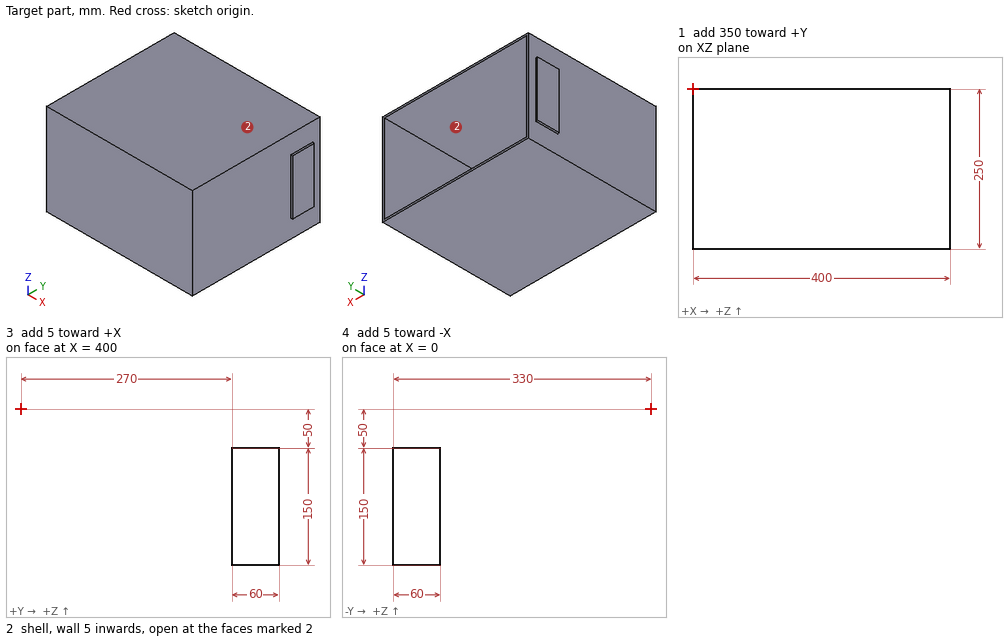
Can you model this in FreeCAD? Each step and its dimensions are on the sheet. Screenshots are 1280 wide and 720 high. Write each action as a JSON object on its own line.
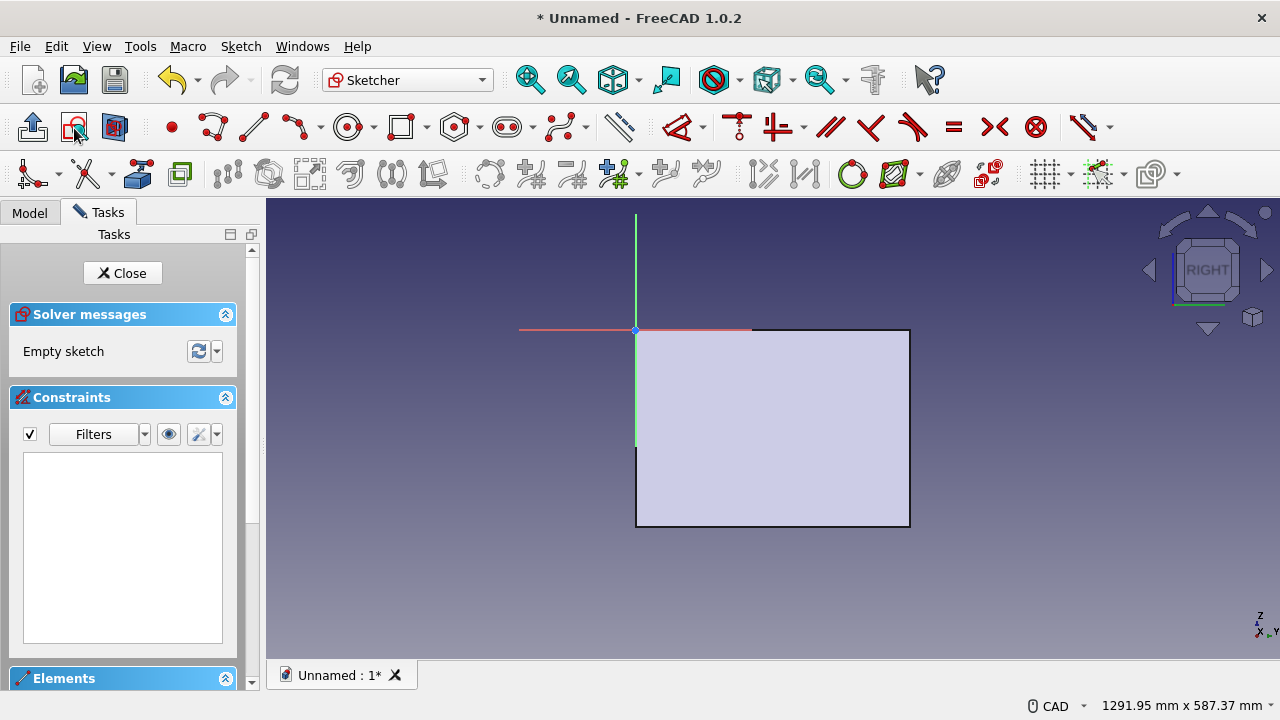
{"action": "scroll", "coordinate": [839, 385], "scroll_direction": "up", "scroll_amount": 3}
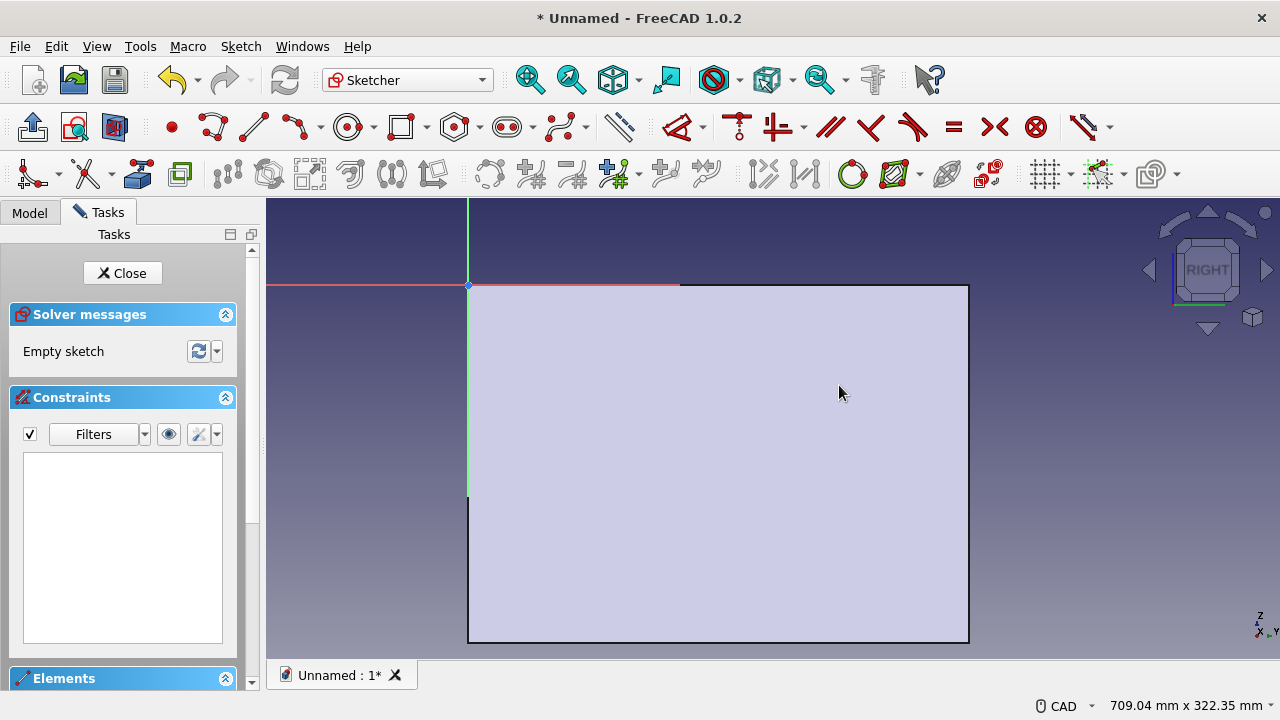
{"action": "left_click", "coordinate": [400, 128]}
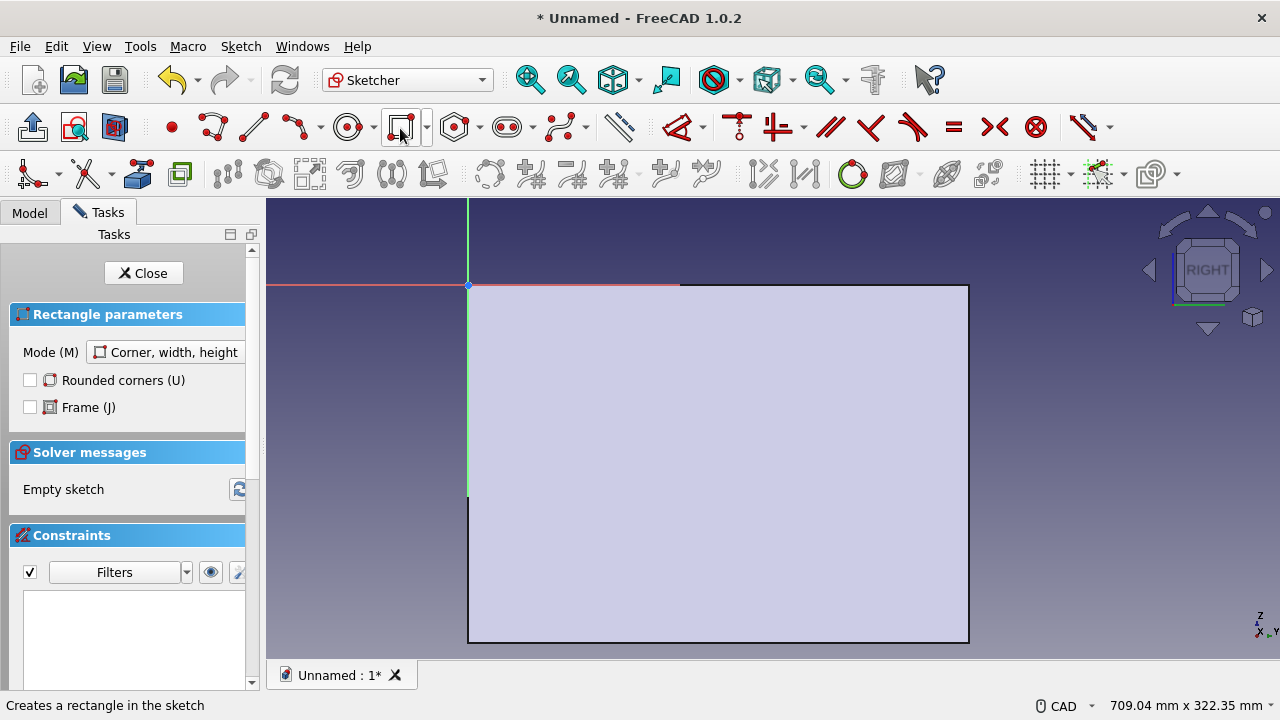
{"action": "left_click", "coordinate": [854, 357]}
{"action": "mouse_move", "coordinate": [940, 571]}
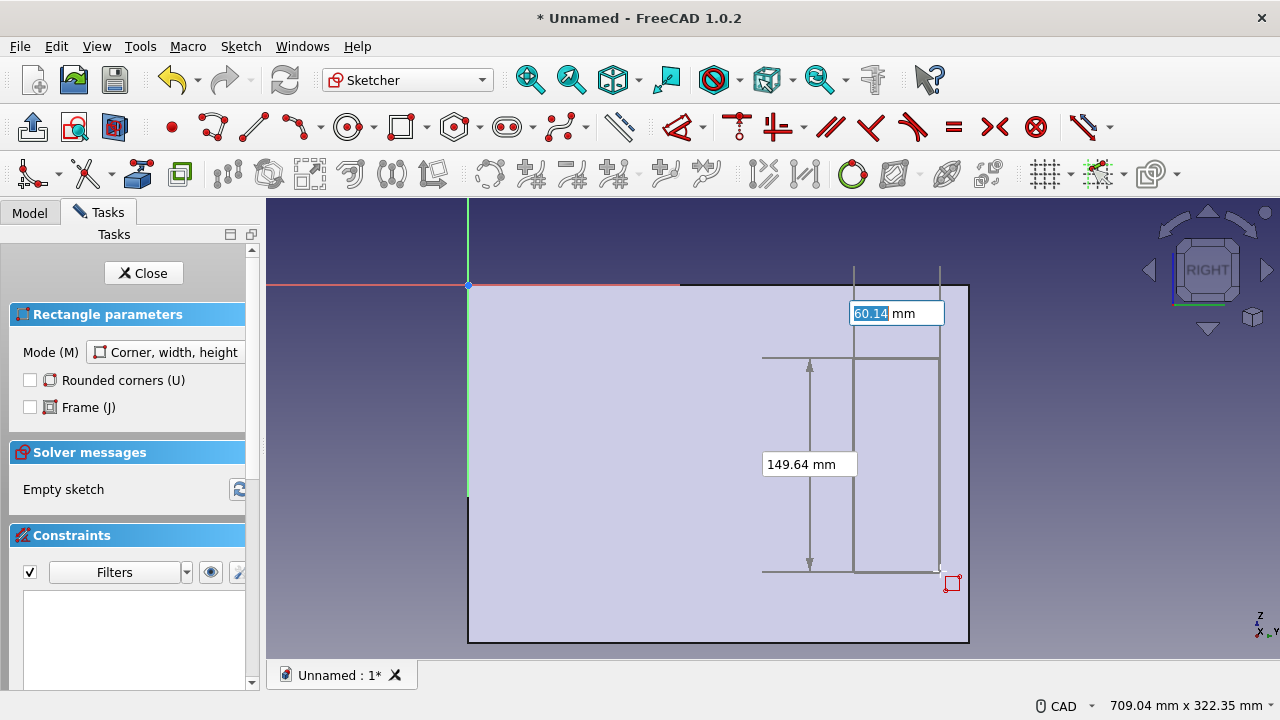
{"action": "type", "text": "60"}
{"action": "key", "text": "Tab"}
{"action": "type", "text": "150"}
{"action": "key", "text": "Return"}
{"action": "key", "text": "Escape"}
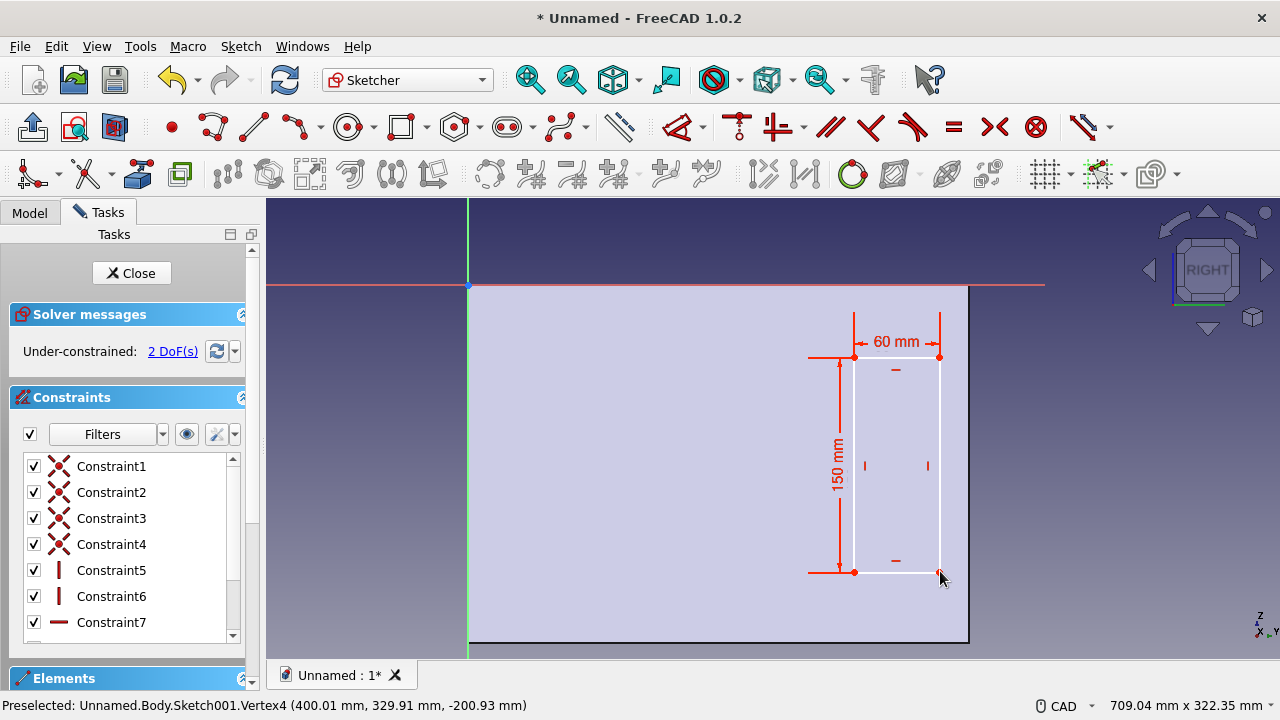
{"action": "key", "text": "d"}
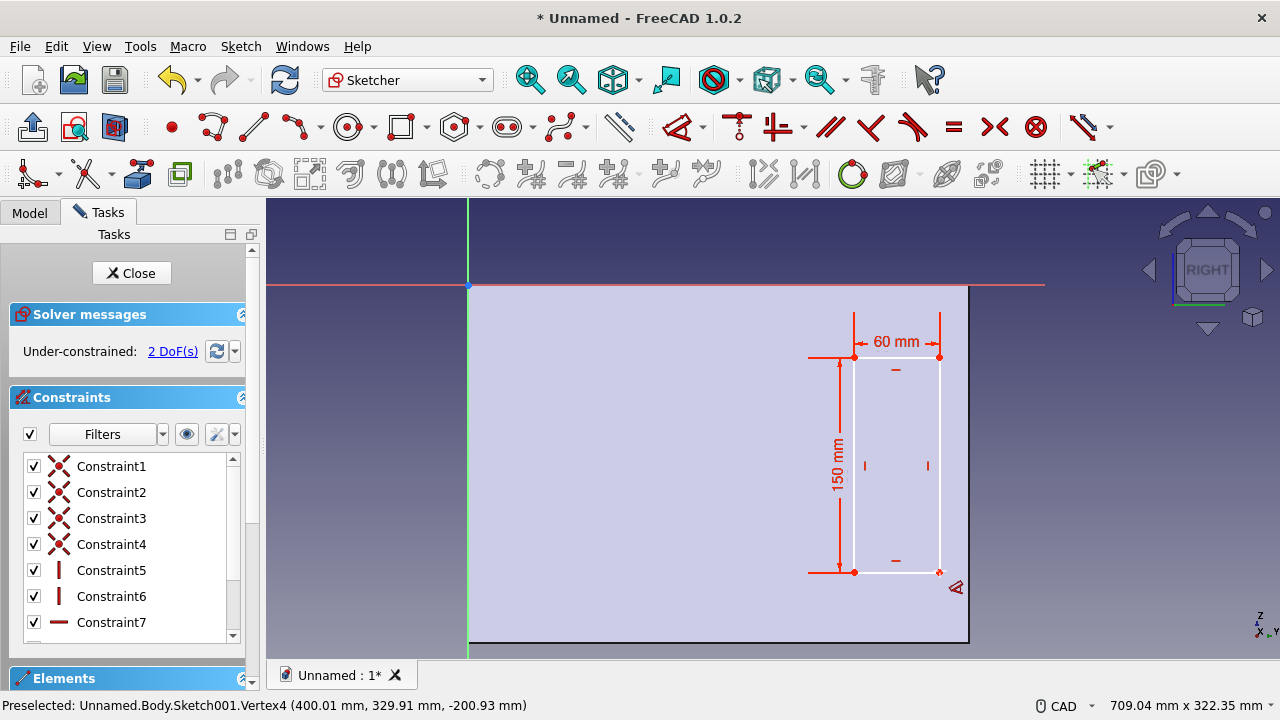
{"action": "left_click", "coordinate": [854, 358]}
{"action": "left_click", "coordinate": [434, 322]}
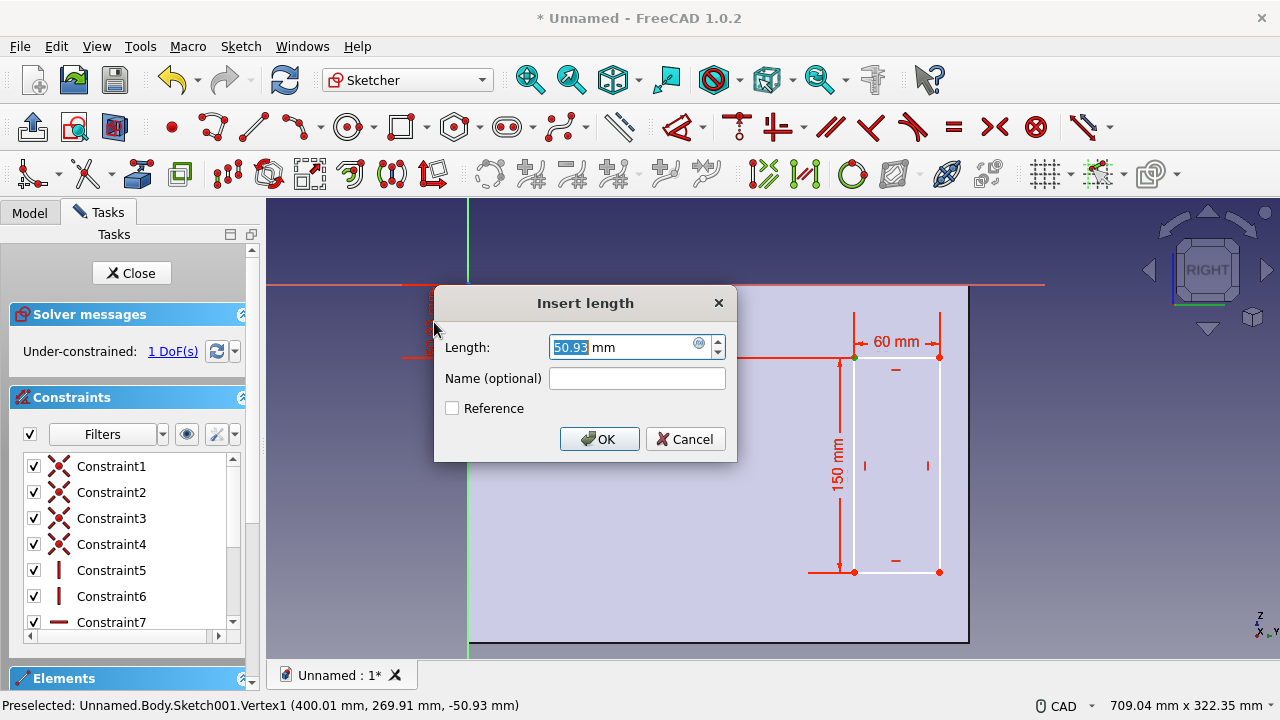
{"action": "type", "text": "50"}
{"action": "key", "text": "Return"}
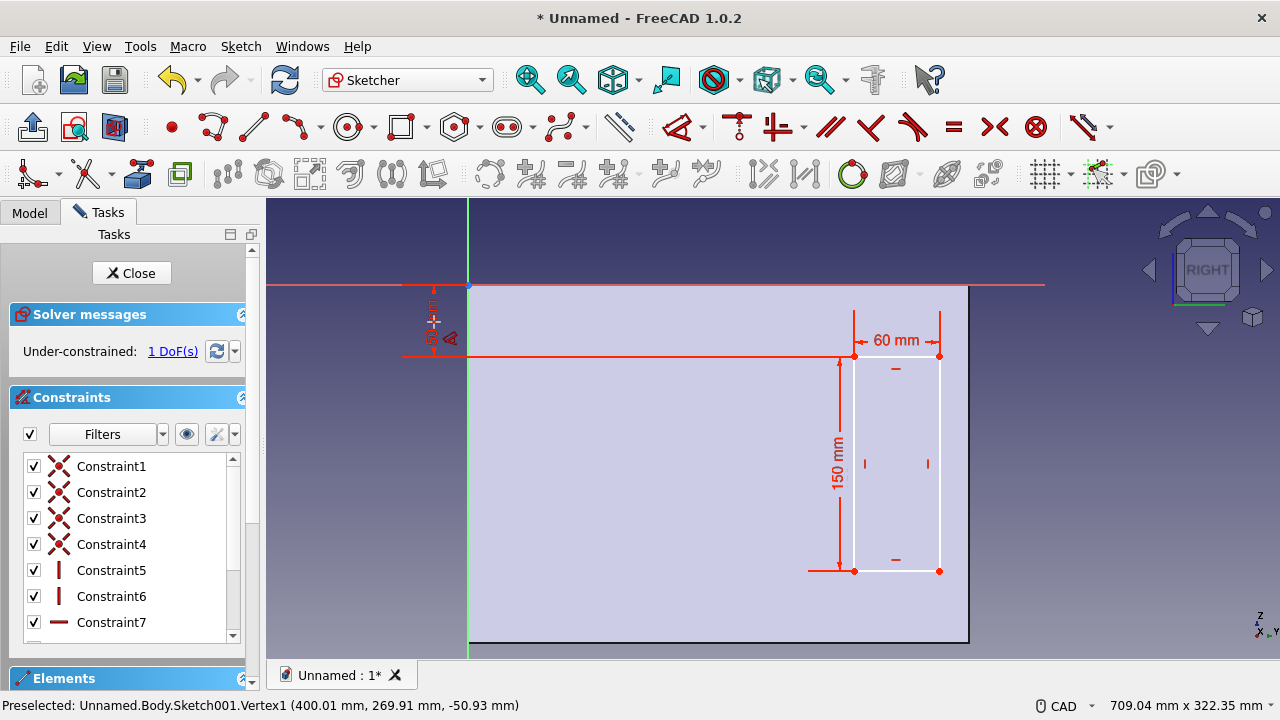
{"action": "left_click", "coordinate": [854, 357]}
{"action": "left_click", "coordinate": [661, 251]}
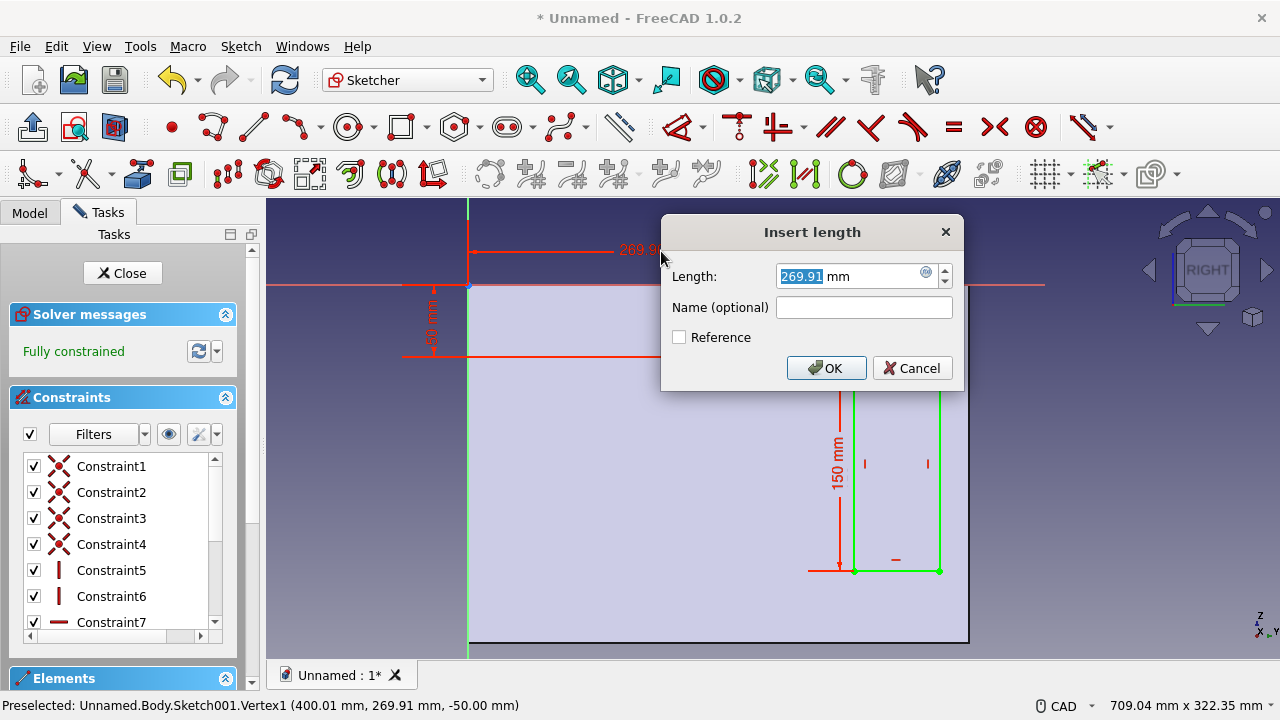
{"action": "type", "text": "270"}
{"action": "key", "text": "Return"}
{"action": "key", "text": "Escape"}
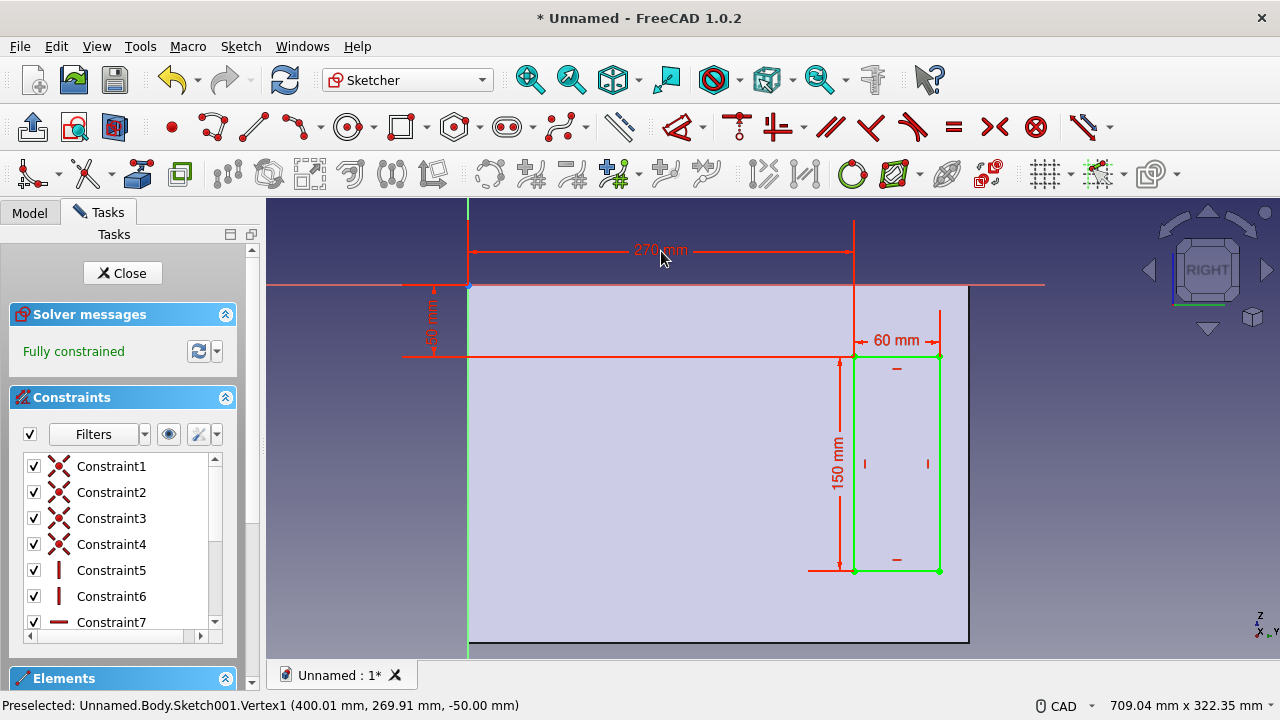
{"action": "left_click", "coordinate": [123, 273]}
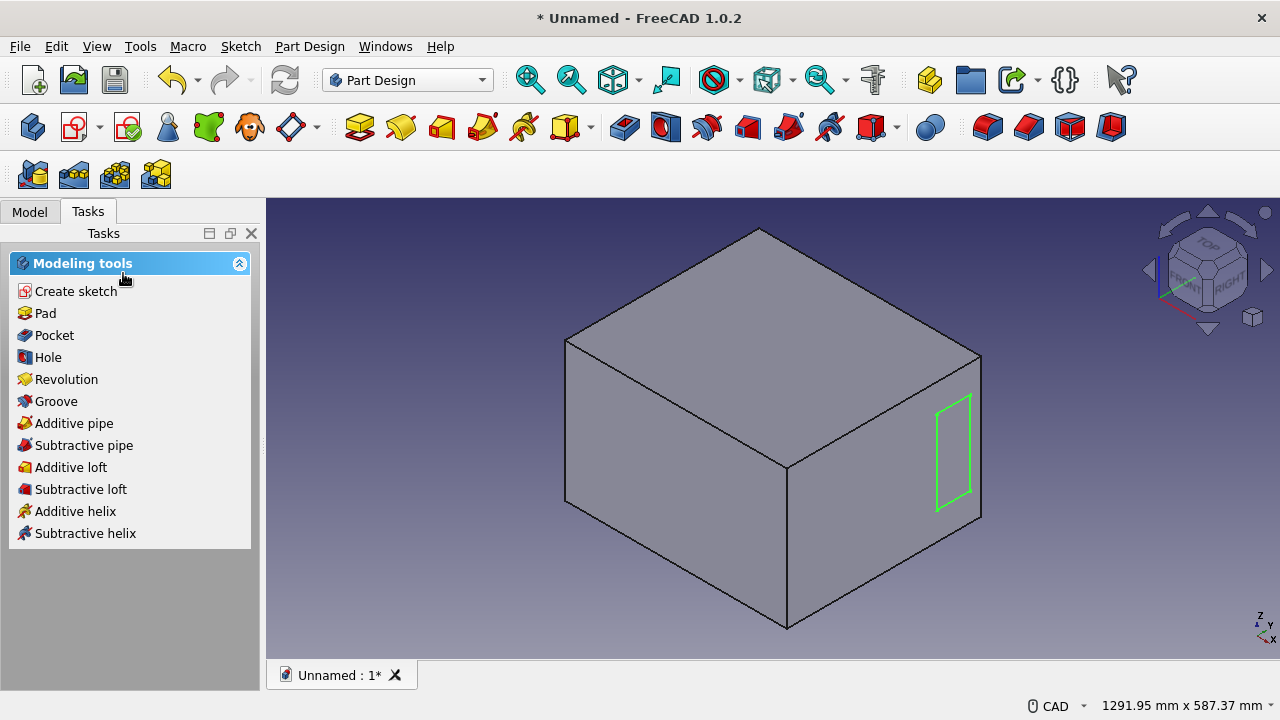
{"action": "left_click", "coordinate": [360, 128]}